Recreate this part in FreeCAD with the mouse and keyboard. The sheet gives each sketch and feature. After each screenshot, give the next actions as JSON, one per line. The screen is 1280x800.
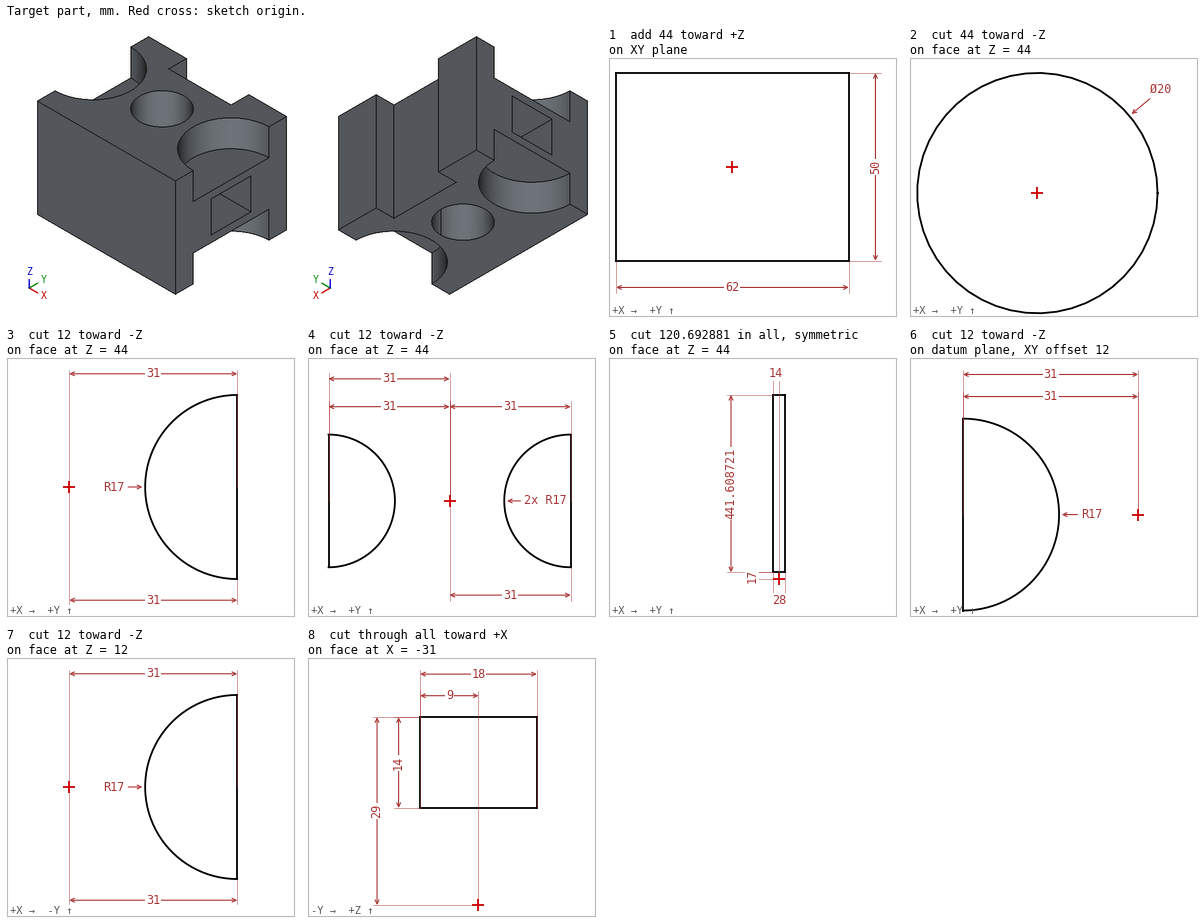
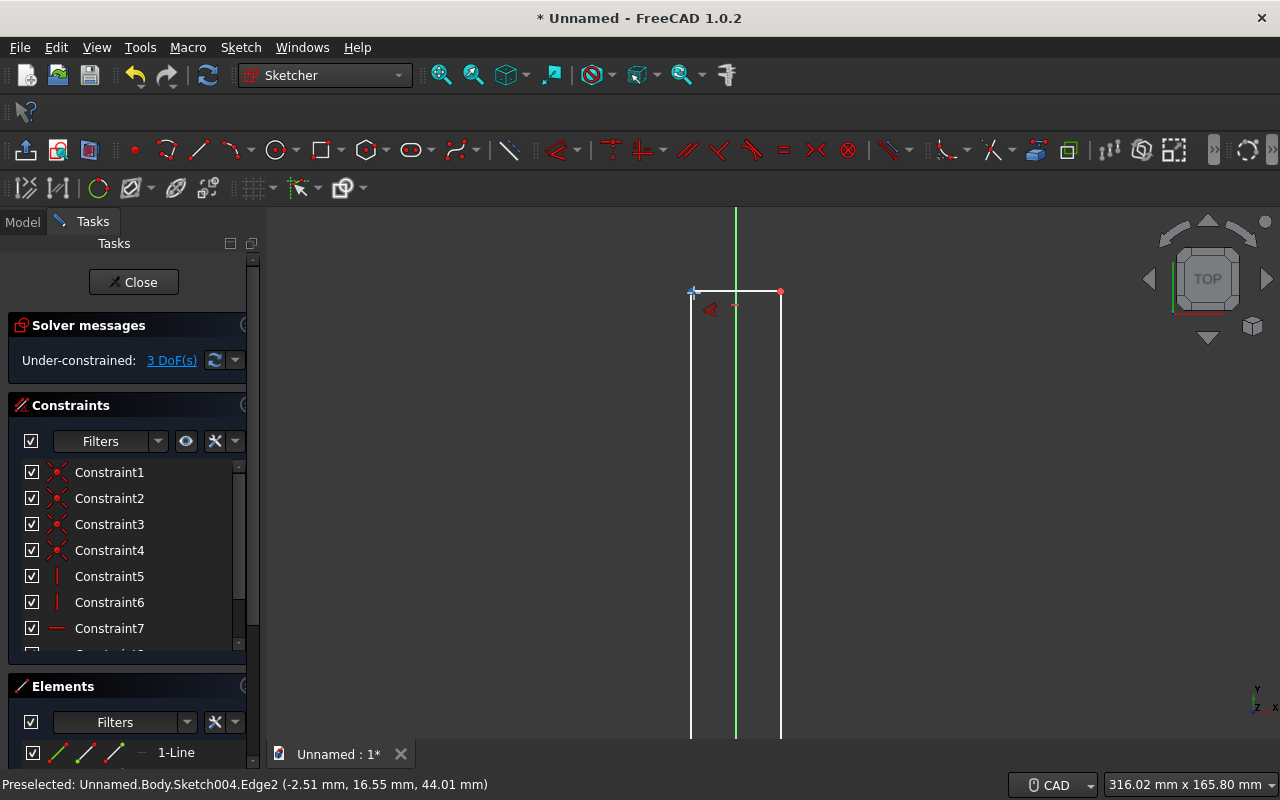
{"action": "left_click", "coordinate": [691, 291]}
{"action": "left_click", "coordinate": [714, 257]}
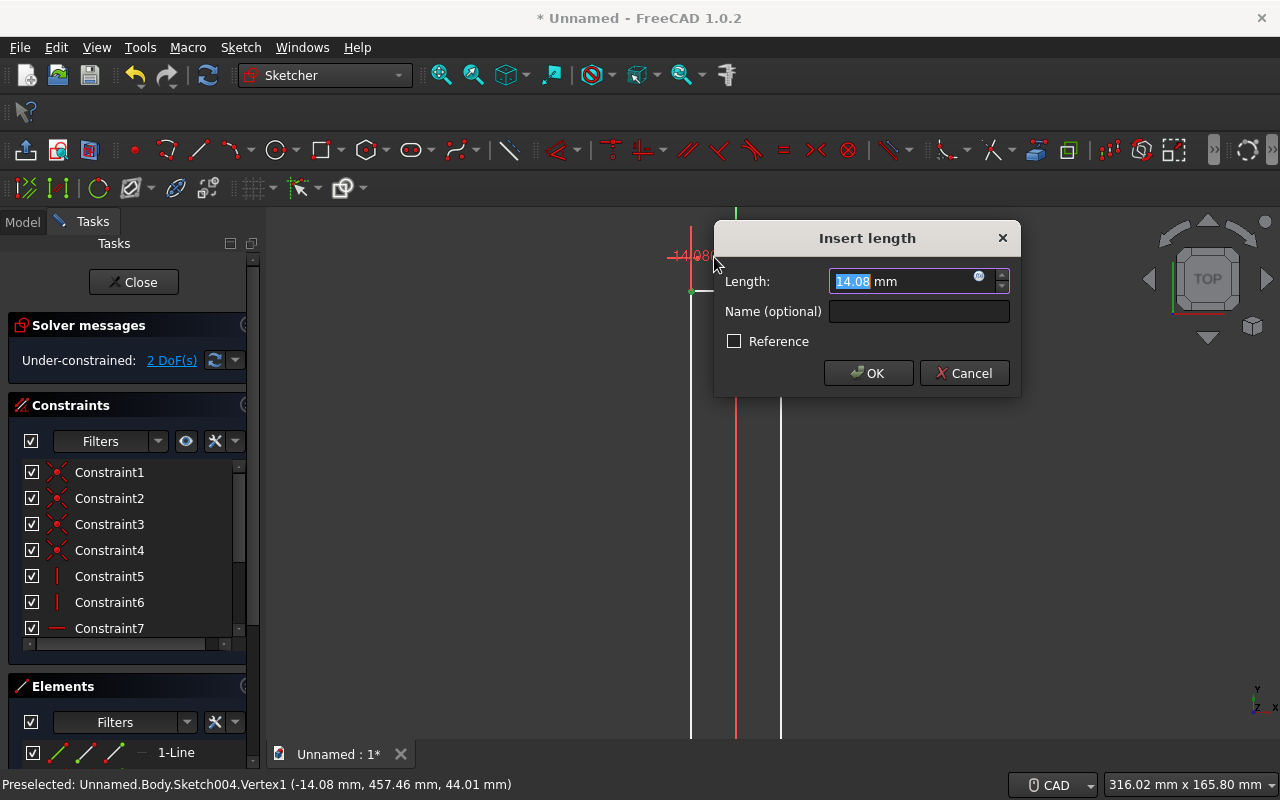
{"action": "type", "text": "14"}
{"action": "key", "text": "Return"}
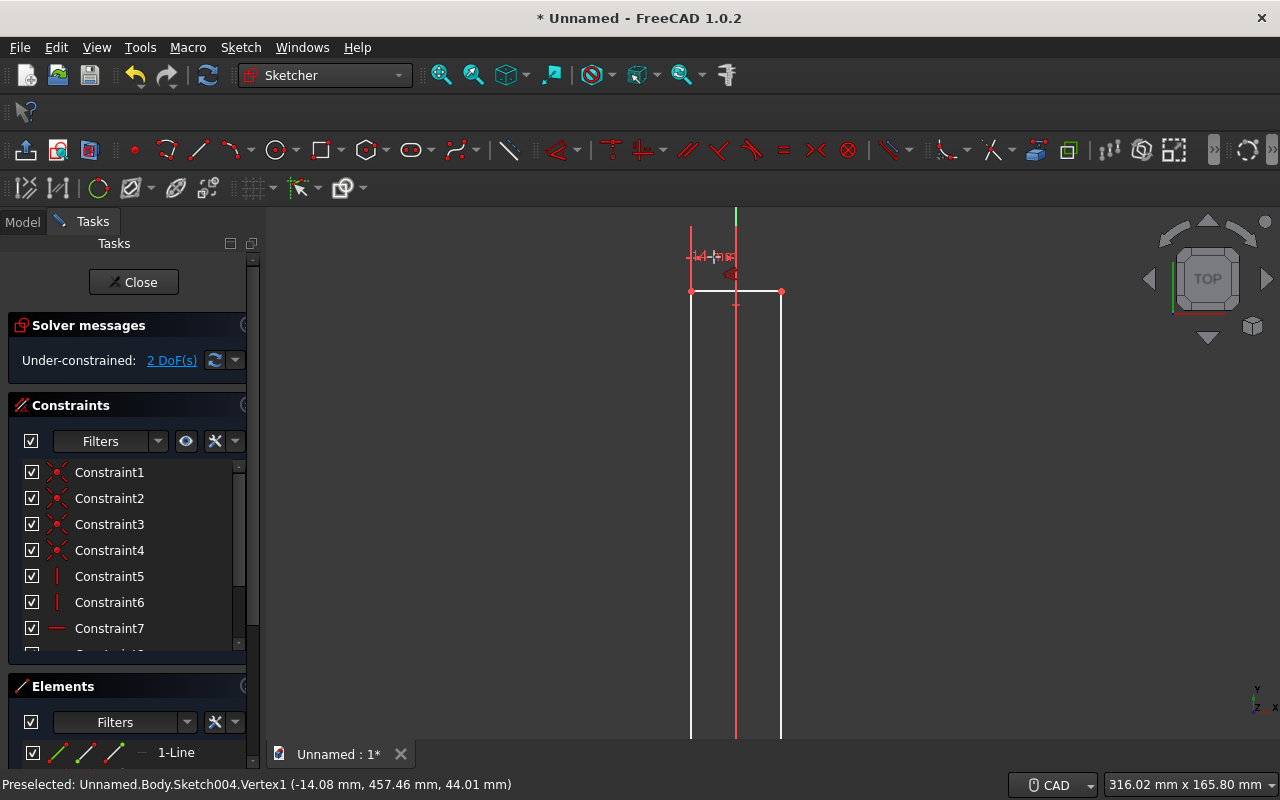
{"action": "scroll", "coordinate": [694, 293], "scroll_direction": "down", "scroll_amount": 7}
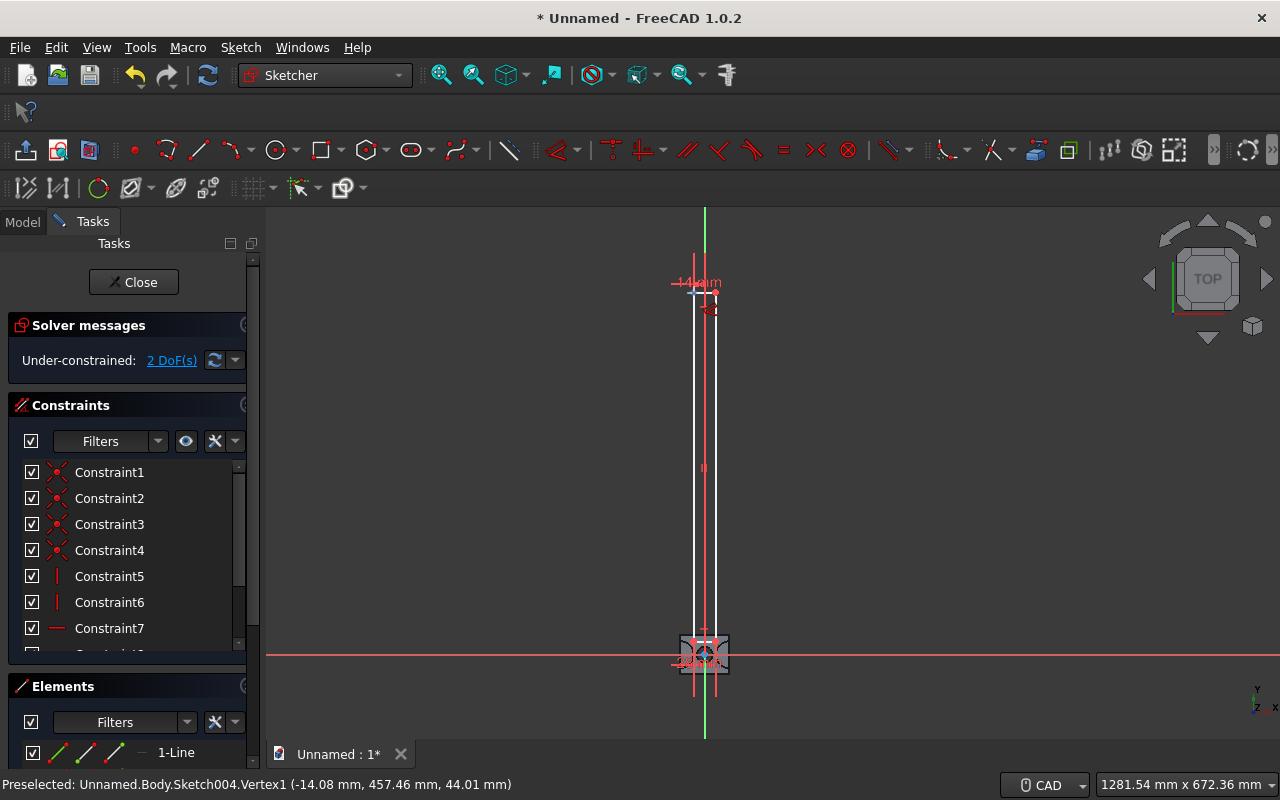
{"action": "scroll", "coordinate": [694, 642], "scroll_direction": "up", "scroll_amount": 6}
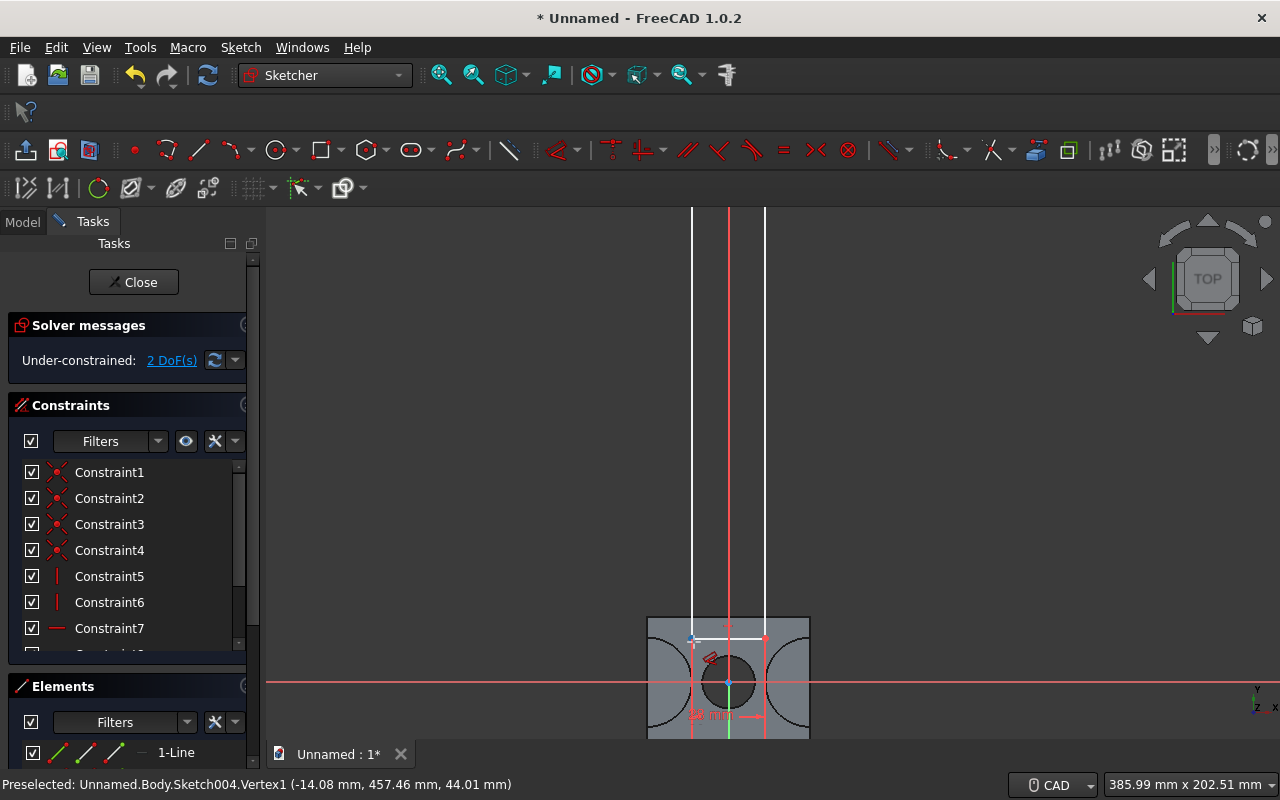
{"action": "left_click", "coordinate": [692, 639]}
{"action": "left_click", "coordinate": [658, 661]}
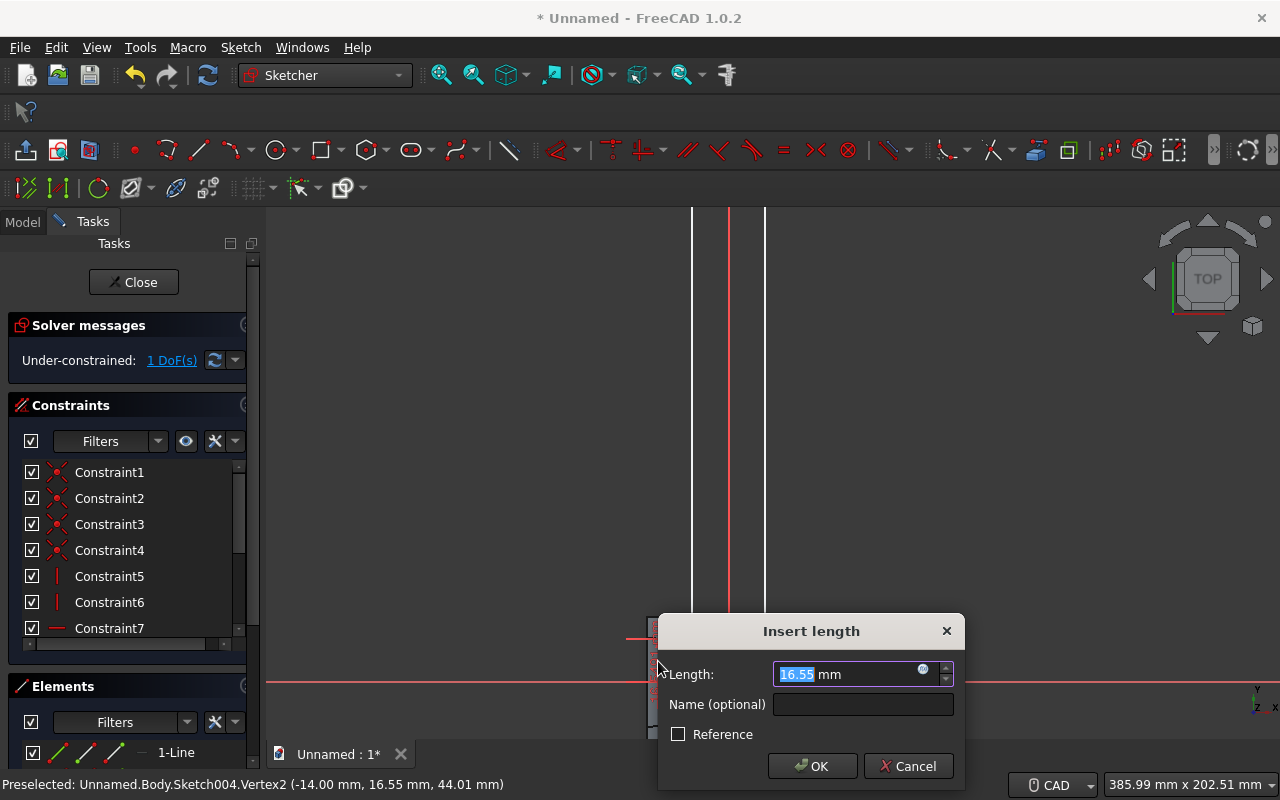
{"action": "type", "text": "17"}
{"action": "key", "text": "Return"}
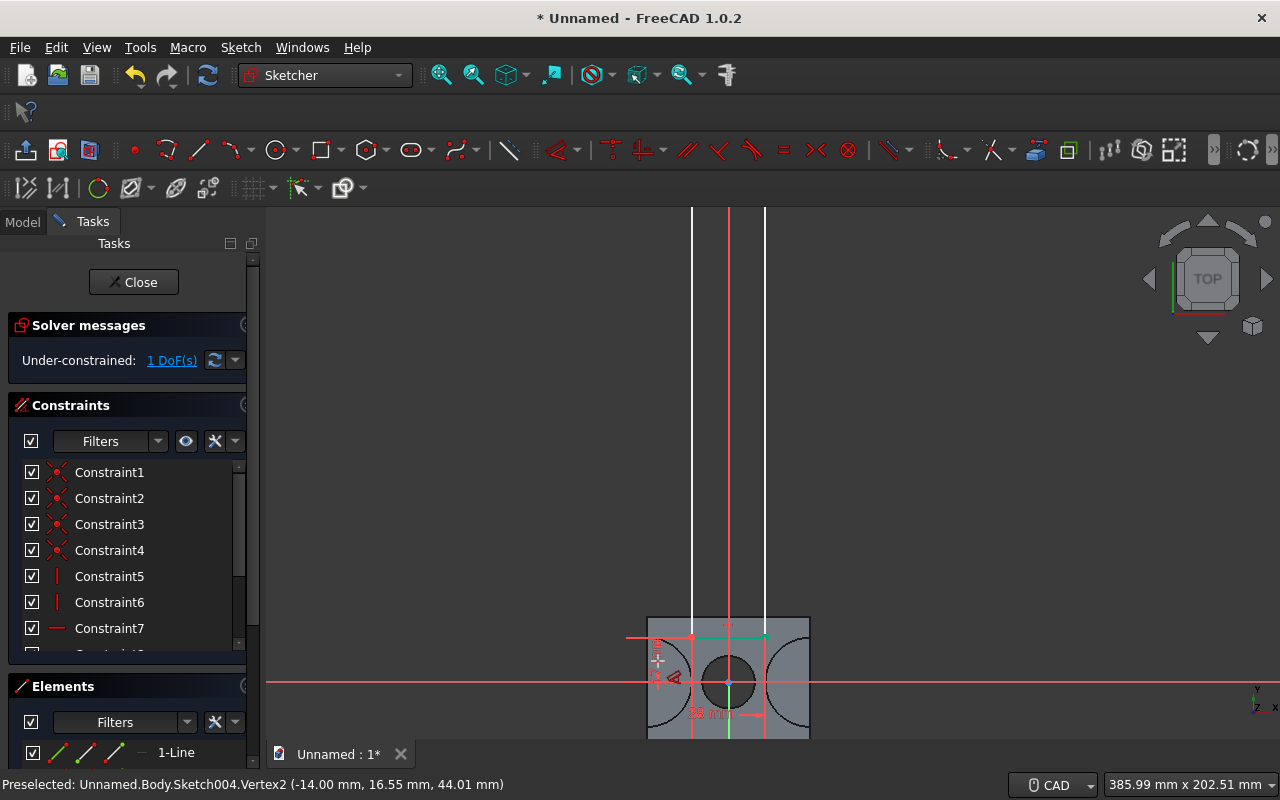
{"action": "left_click", "coordinate": [692, 290]}
{"action": "left_click", "coordinate": [658, 436]}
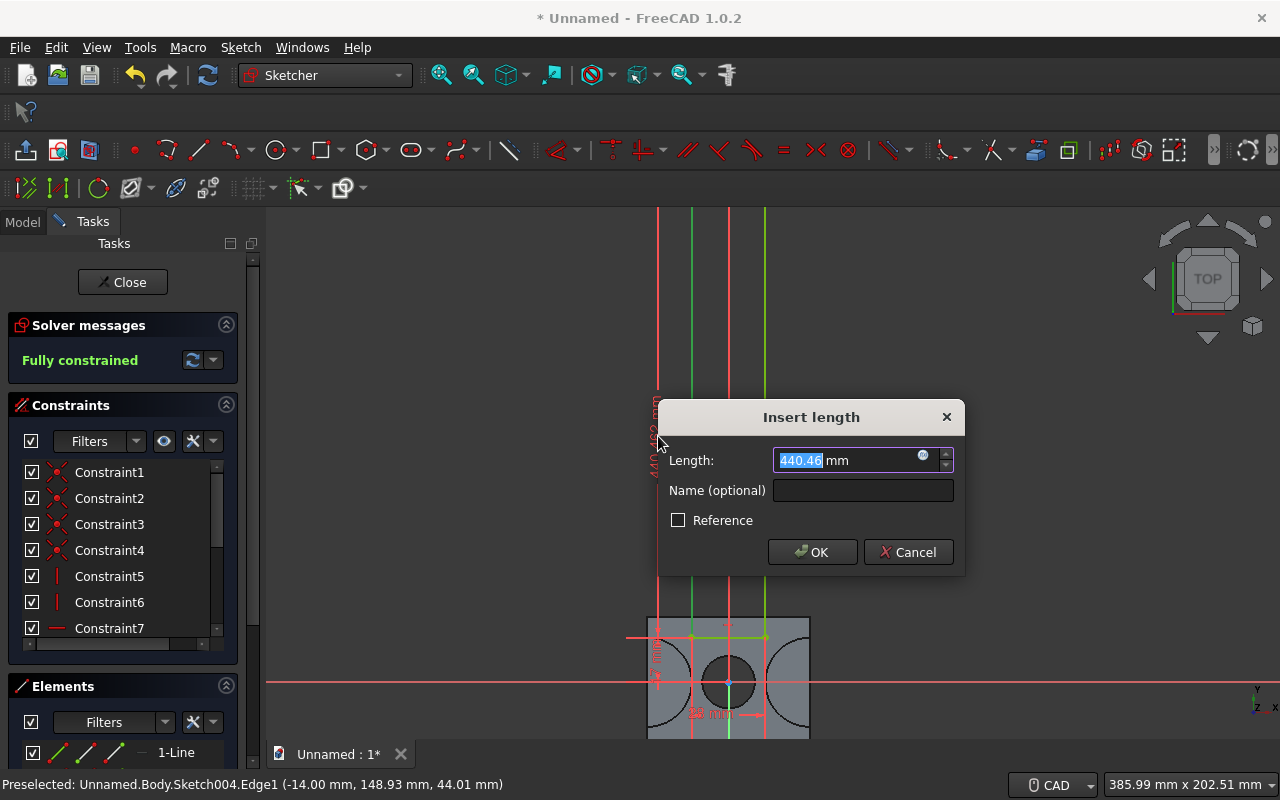
{"action": "type", "text": "441.608721"}
{"action": "key", "text": "Return"}
{"action": "key", "text": "Escape"}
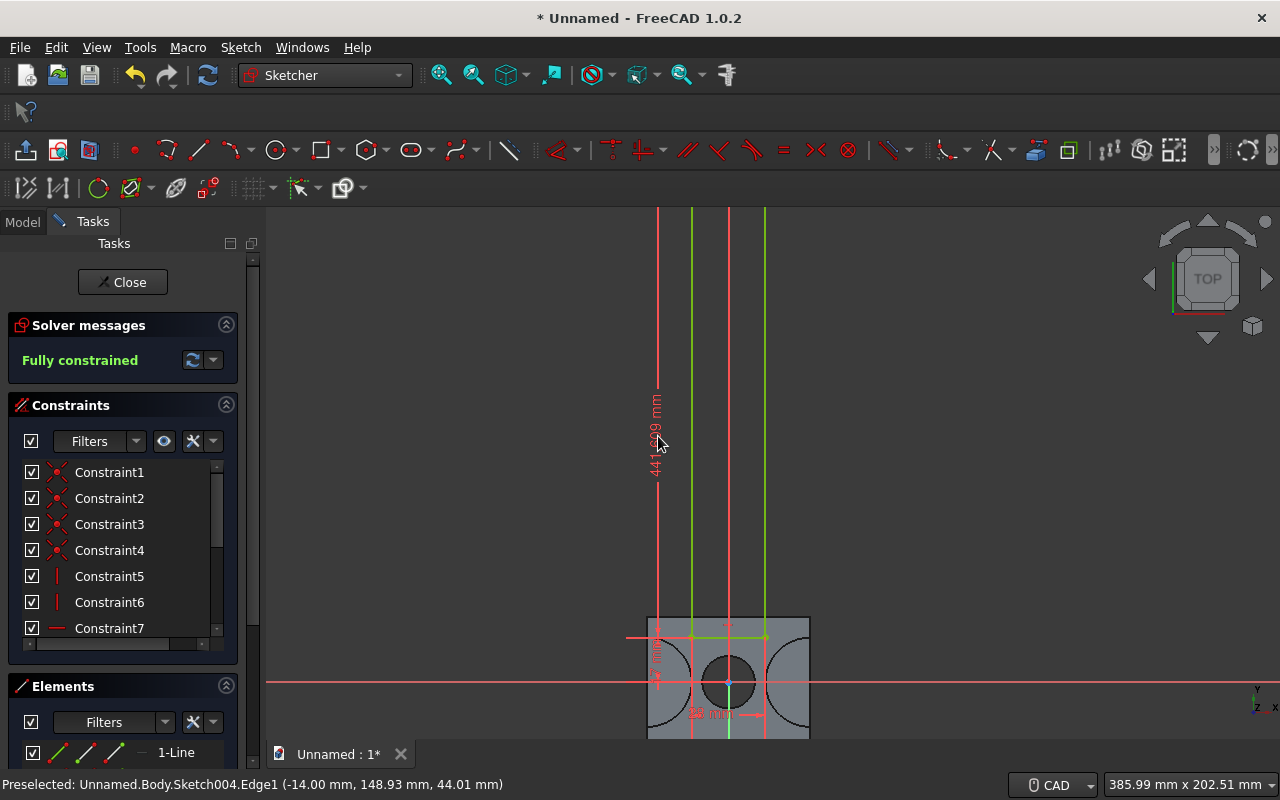
{"action": "left_click", "coordinate": [123, 282]}